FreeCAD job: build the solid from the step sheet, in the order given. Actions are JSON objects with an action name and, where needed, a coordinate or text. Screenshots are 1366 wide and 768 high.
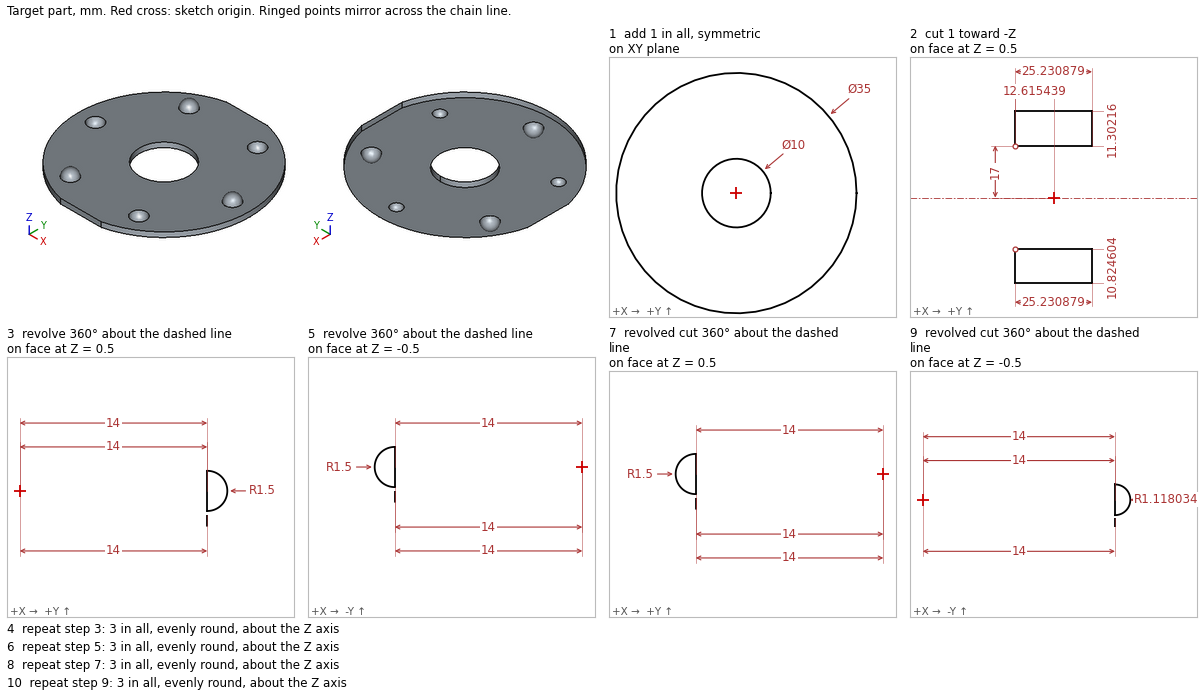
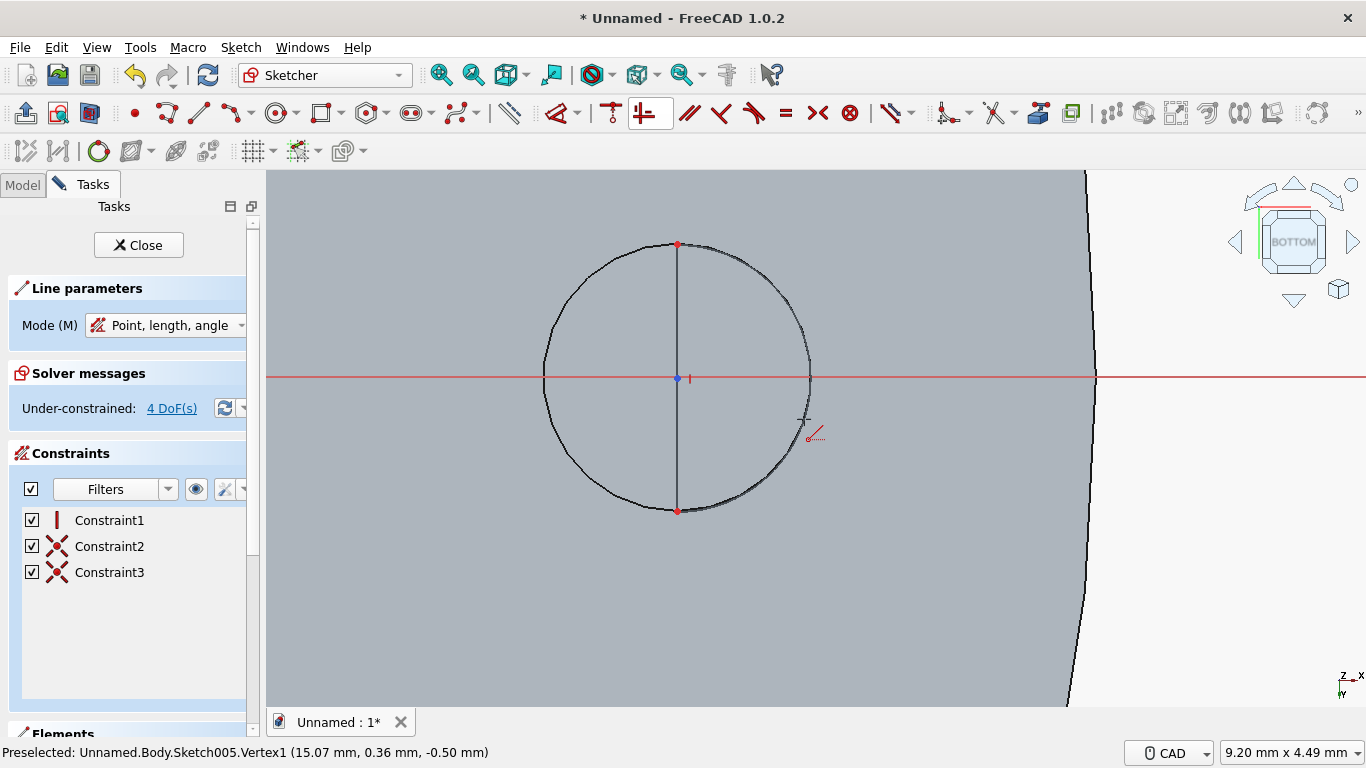
{"action": "left_click", "coordinate": [677, 538]}
{"action": "left_click", "coordinate": [677, 618]}
{"action": "key", "text": "Escape"}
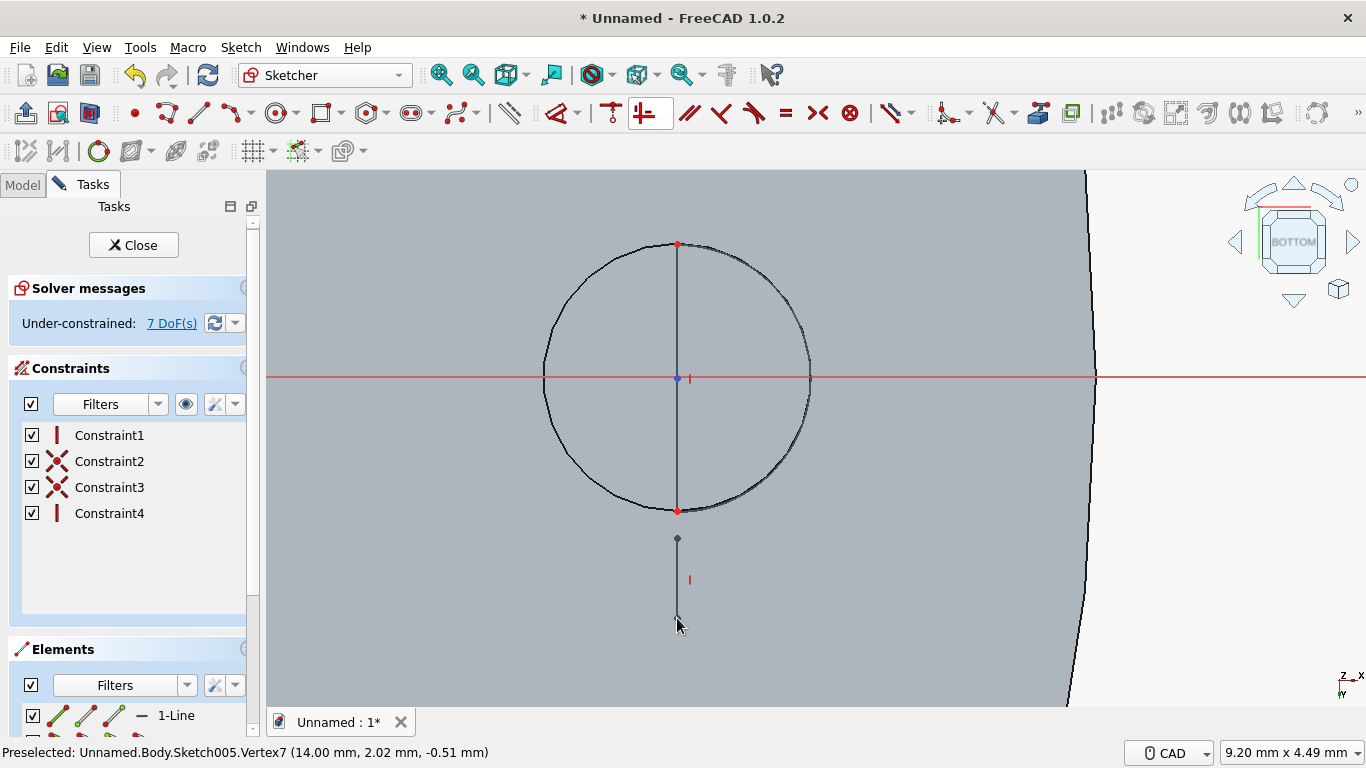
{"action": "left_click", "coordinate": [677, 563]}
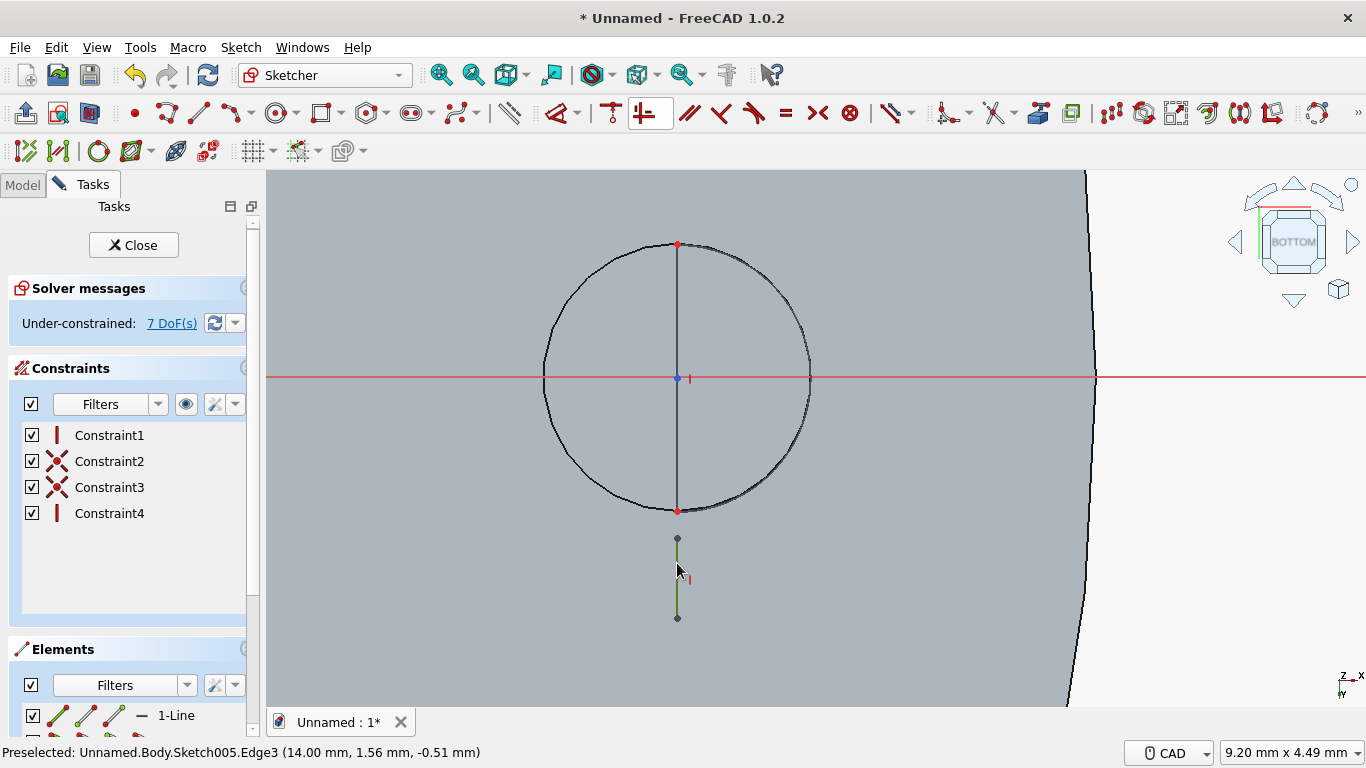
{"action": "left_click", "coordinate": [510, 114]}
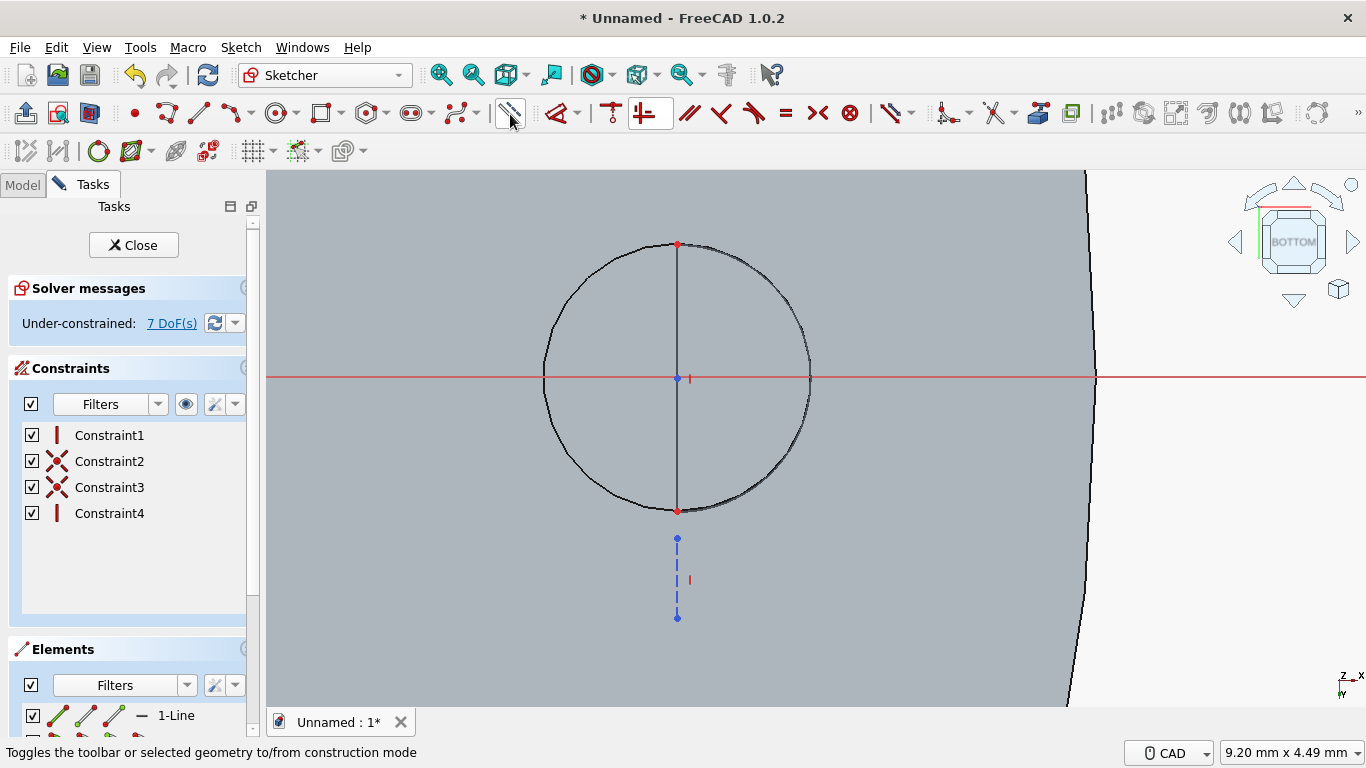
{"action": "left_click", "coordinate": [677, 378]}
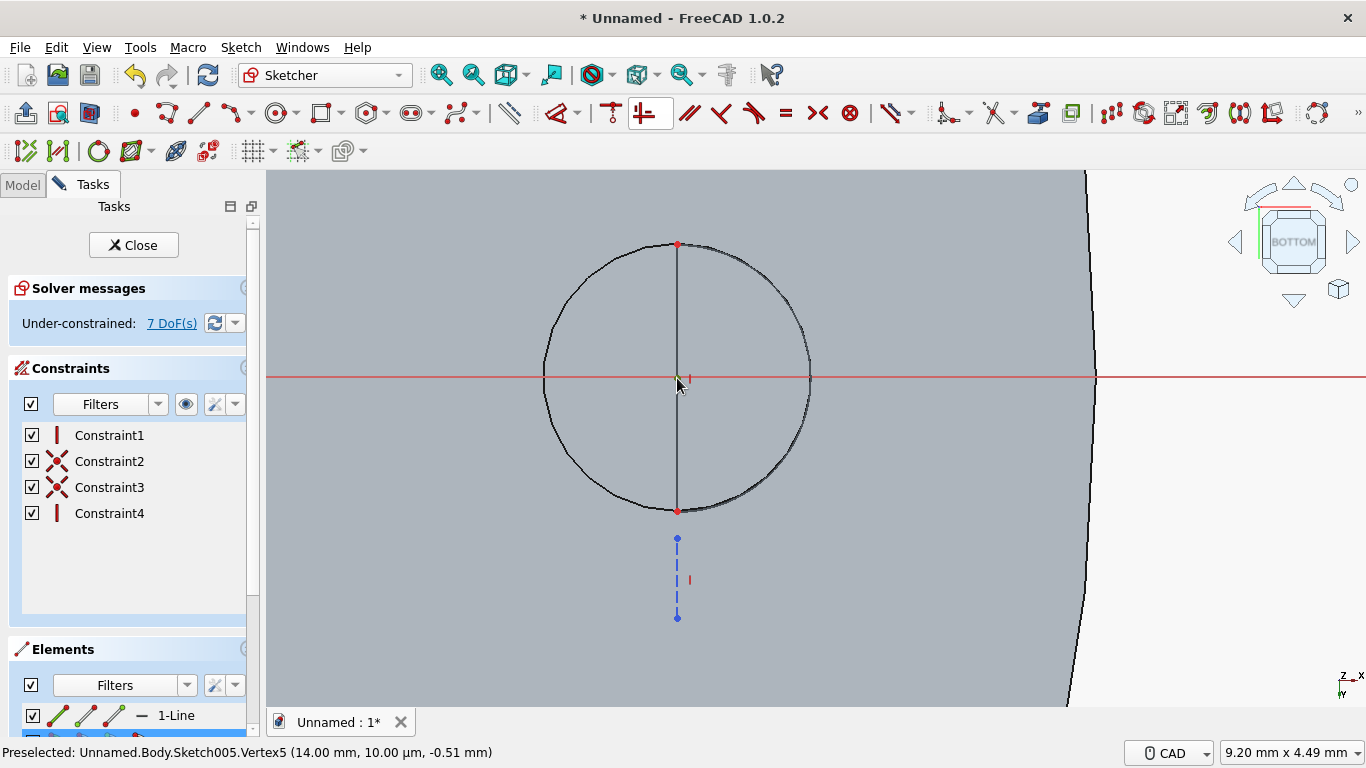
{"action": "left_click", "coordinate": [359, 377]}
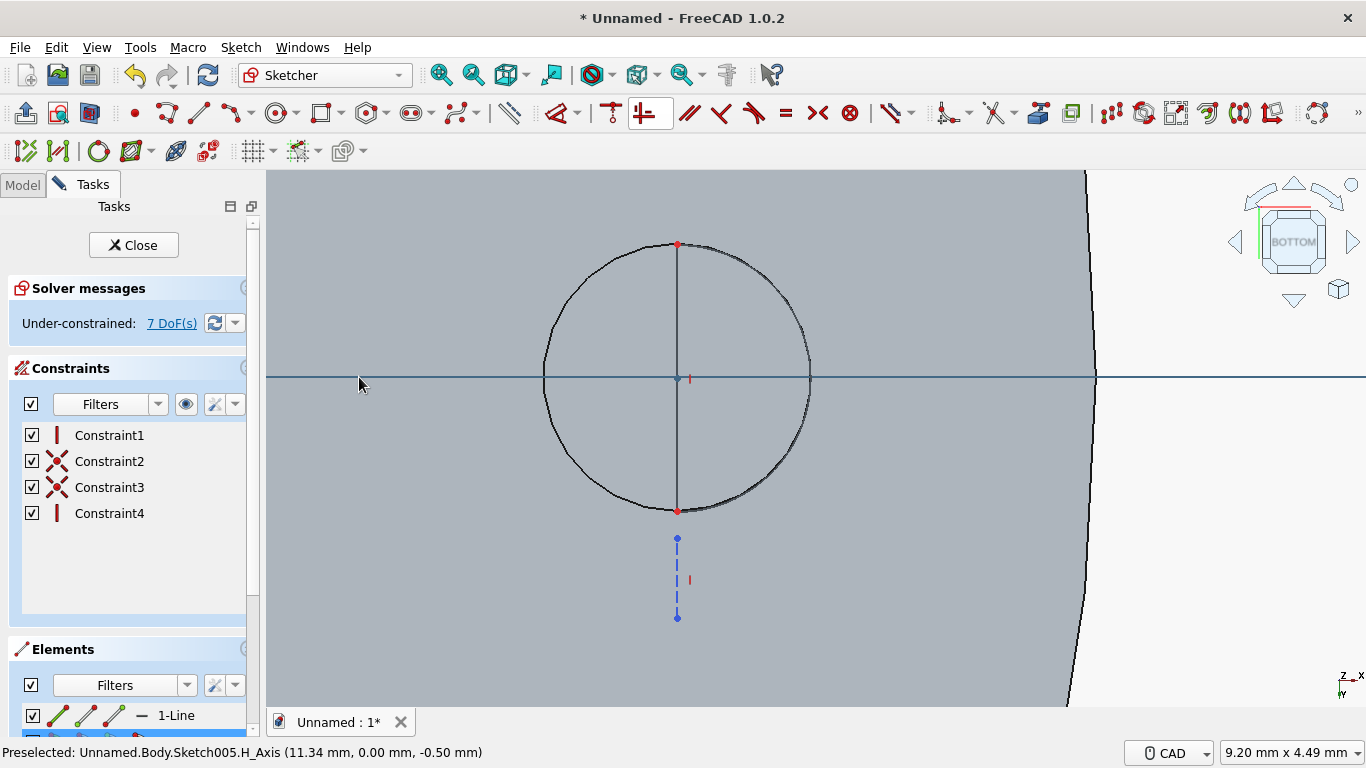
{"action": "key", "text": "c"}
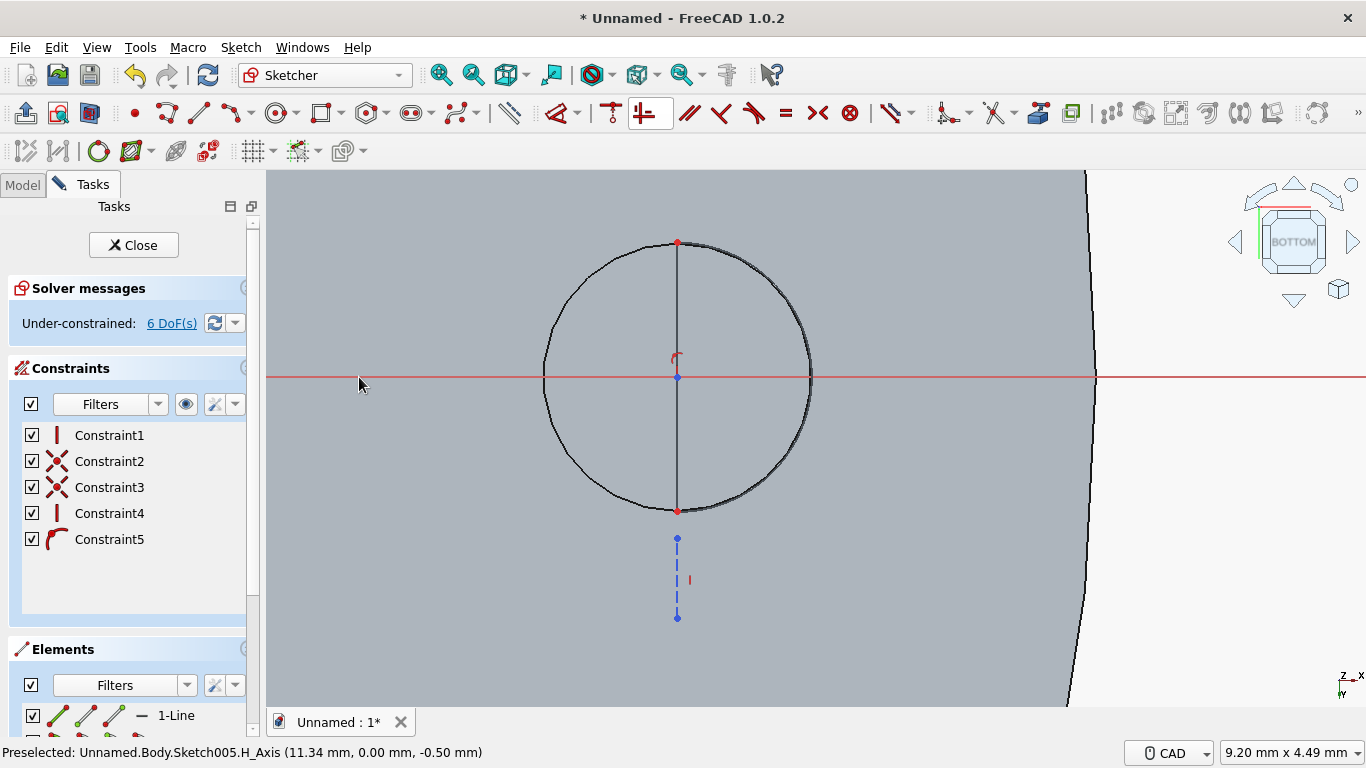
{"action": "key", "text": "d"}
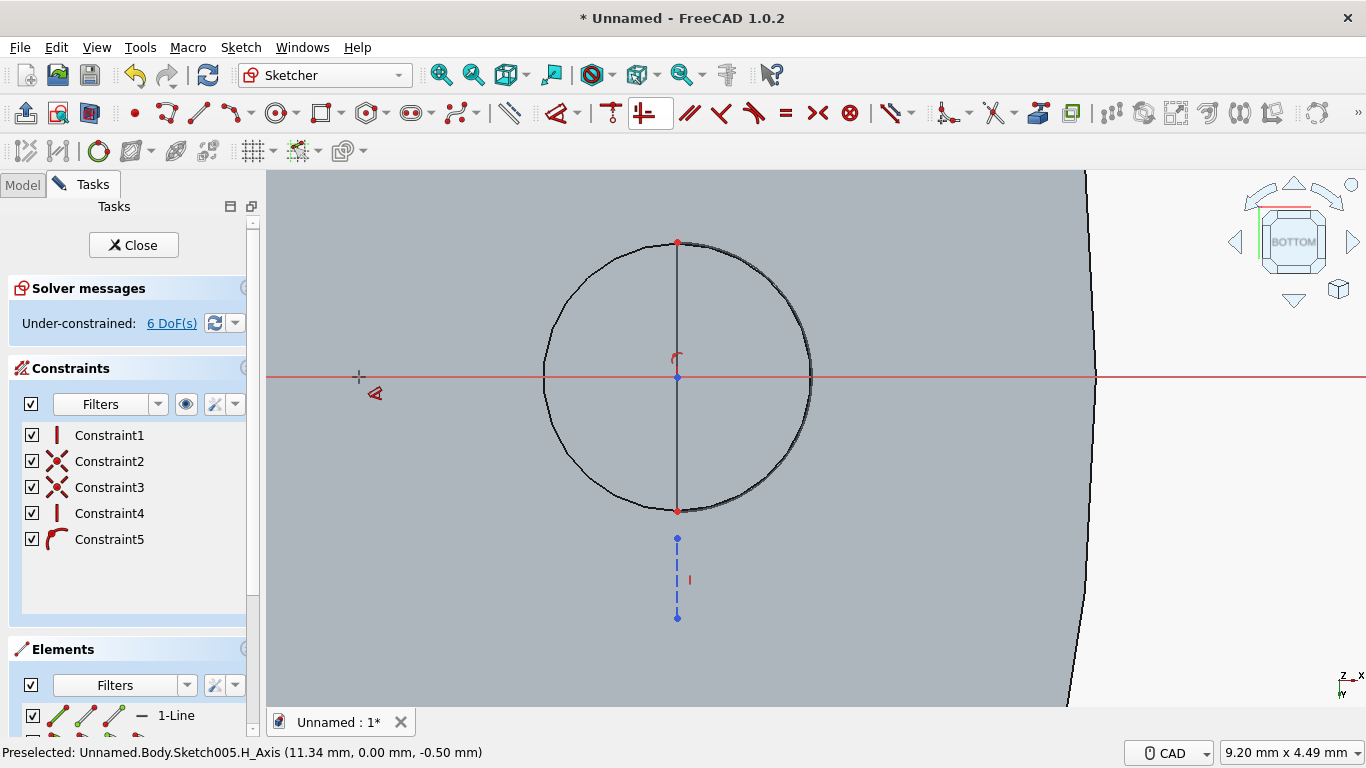
{"action": "left_click", "coordinate": [786, 457]}
{"action": "left_click", "coordinate": [812, 476]}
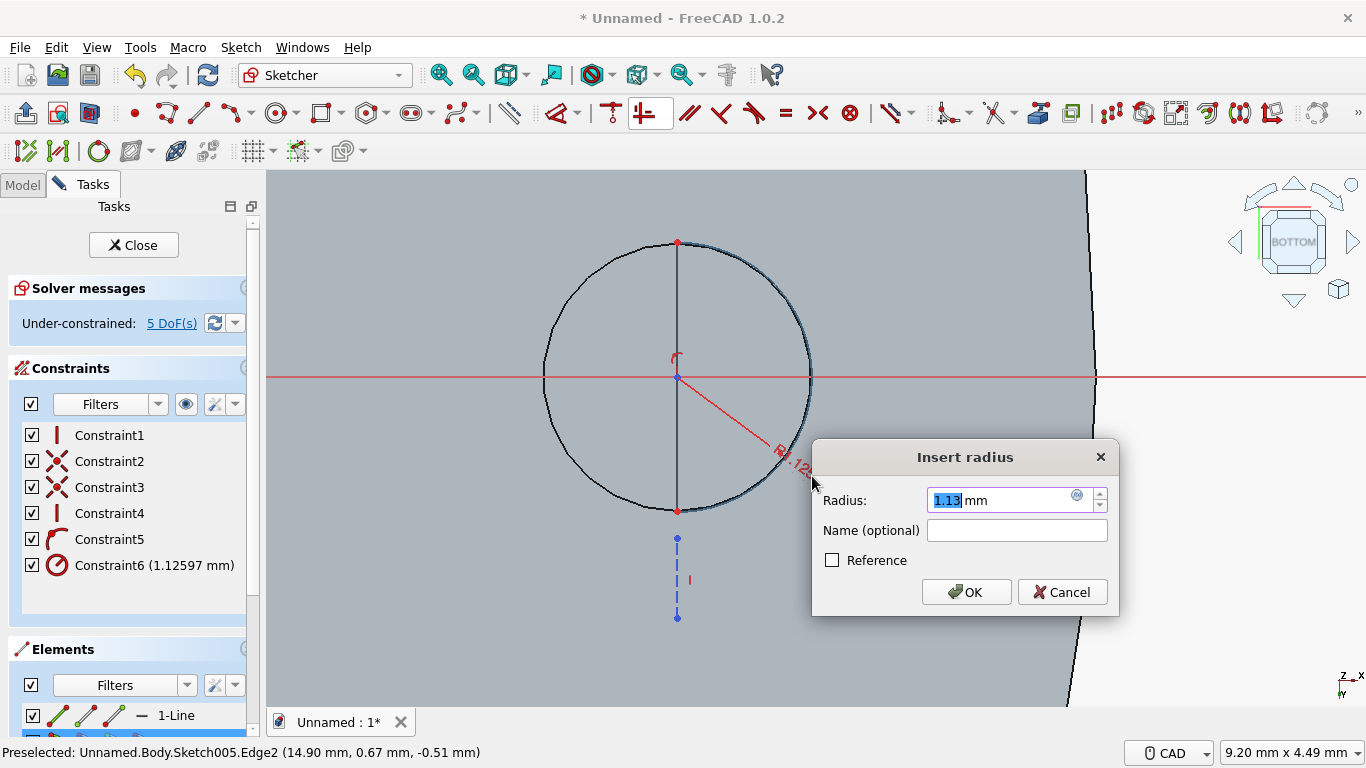
{"action": "type", "text": "1.118034"}
{"action": "key", "text": "Return"}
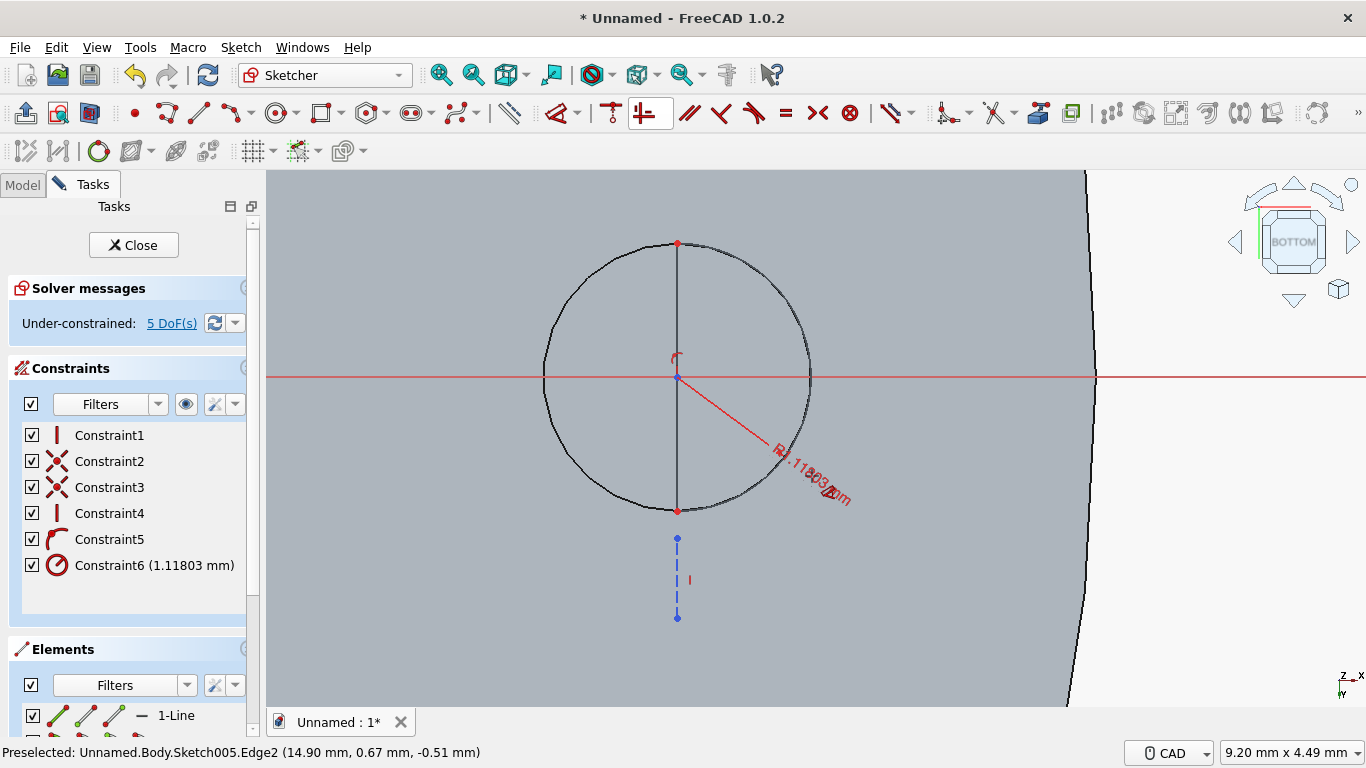
{"action": "left_click", "coordinate": [677, 244]}
{"action": "left_click", "coordinate": [485, 210]}